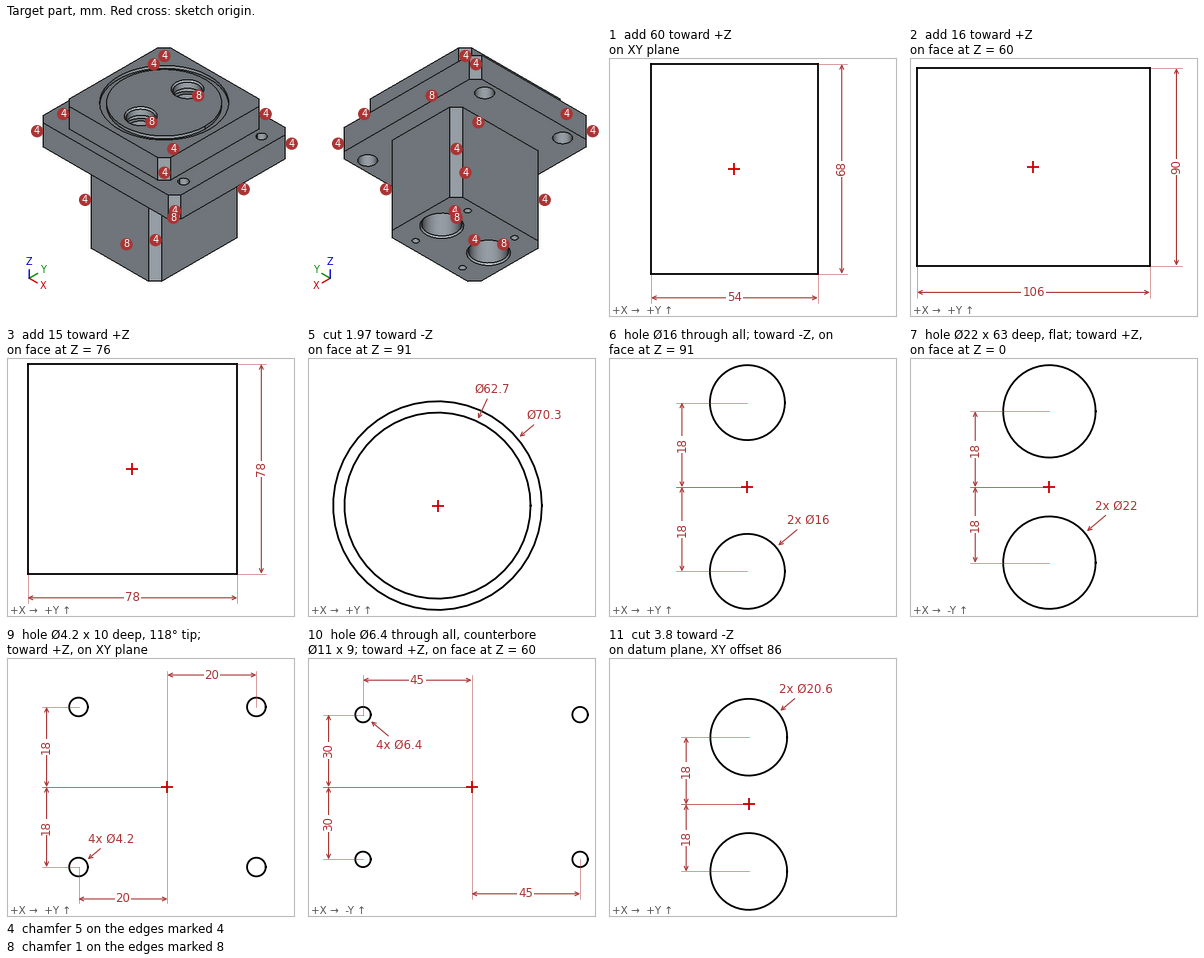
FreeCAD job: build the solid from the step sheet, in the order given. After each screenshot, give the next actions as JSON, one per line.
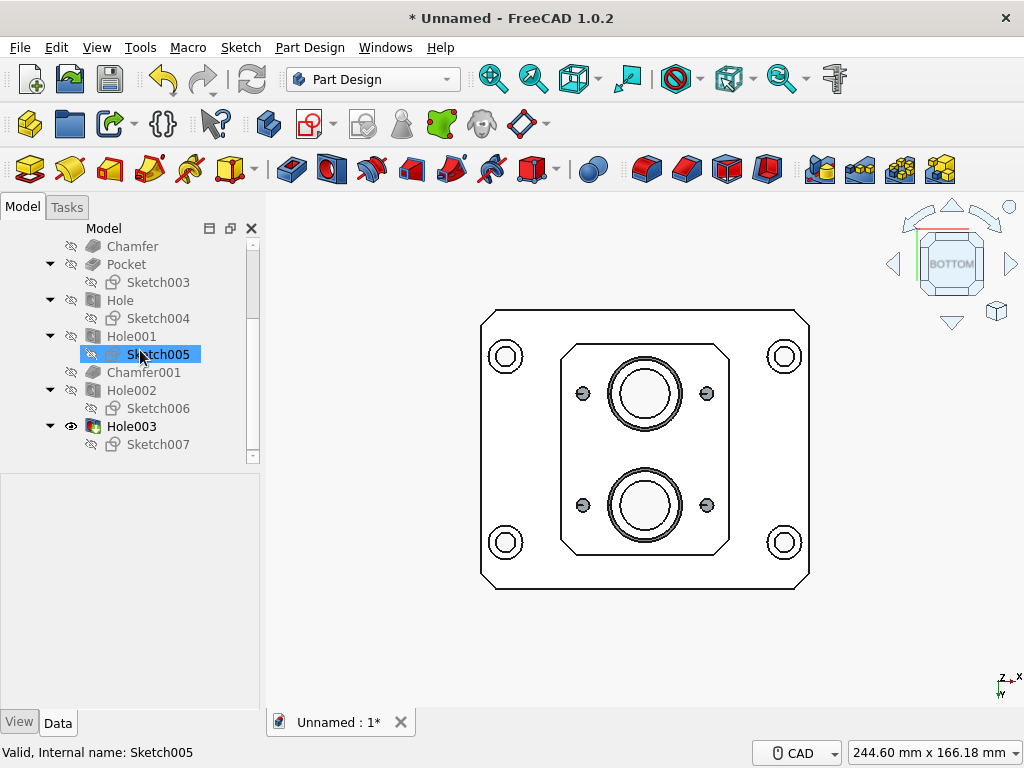
{"action": "scroll", "coordinate": [140, 350], "scroll_direction": "up", "scroll_amount": 15}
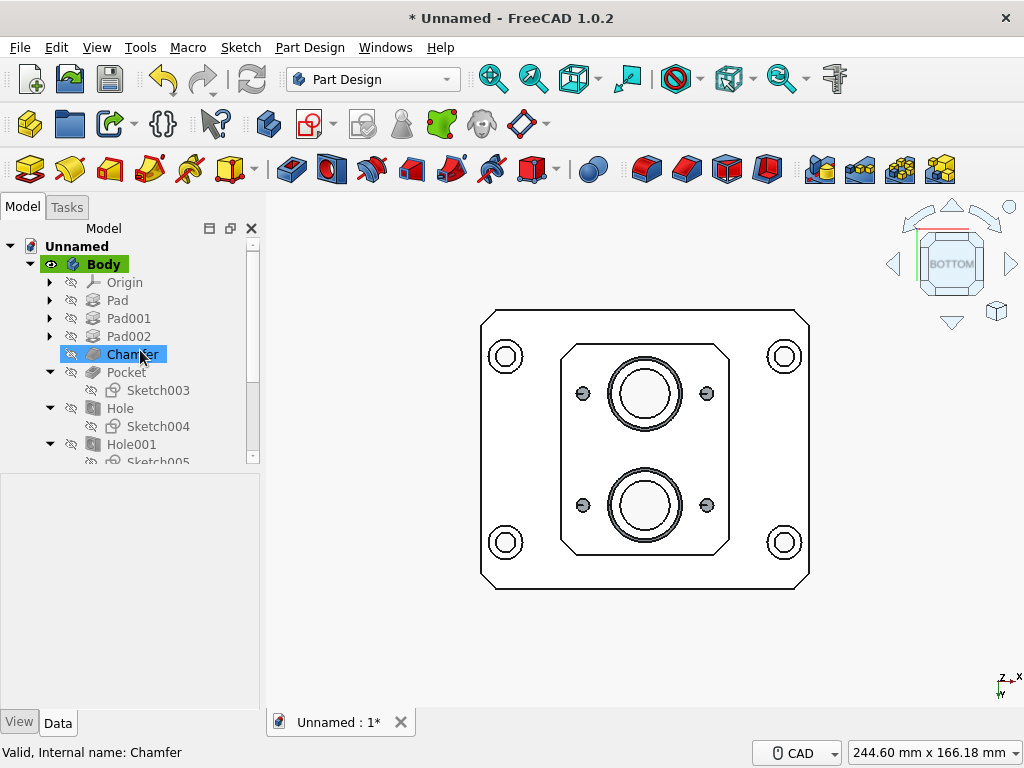
{"action": "left_click", "coordinate": [50, 282]}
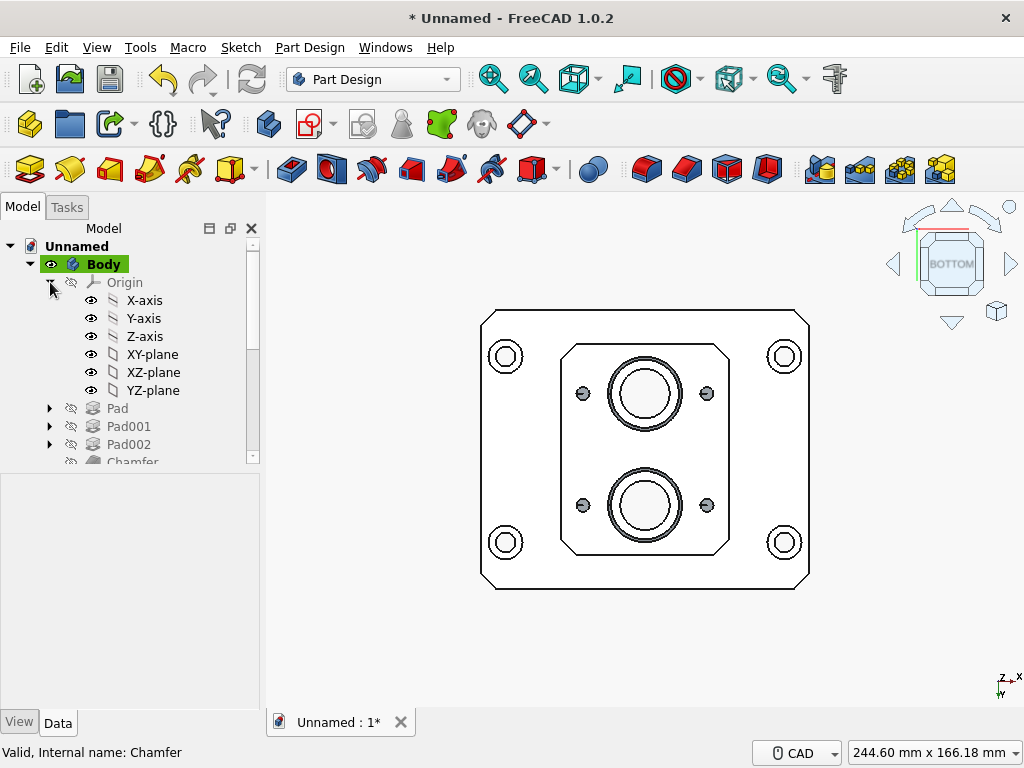
{"action": "left_click", "coordinate": [136, 354]}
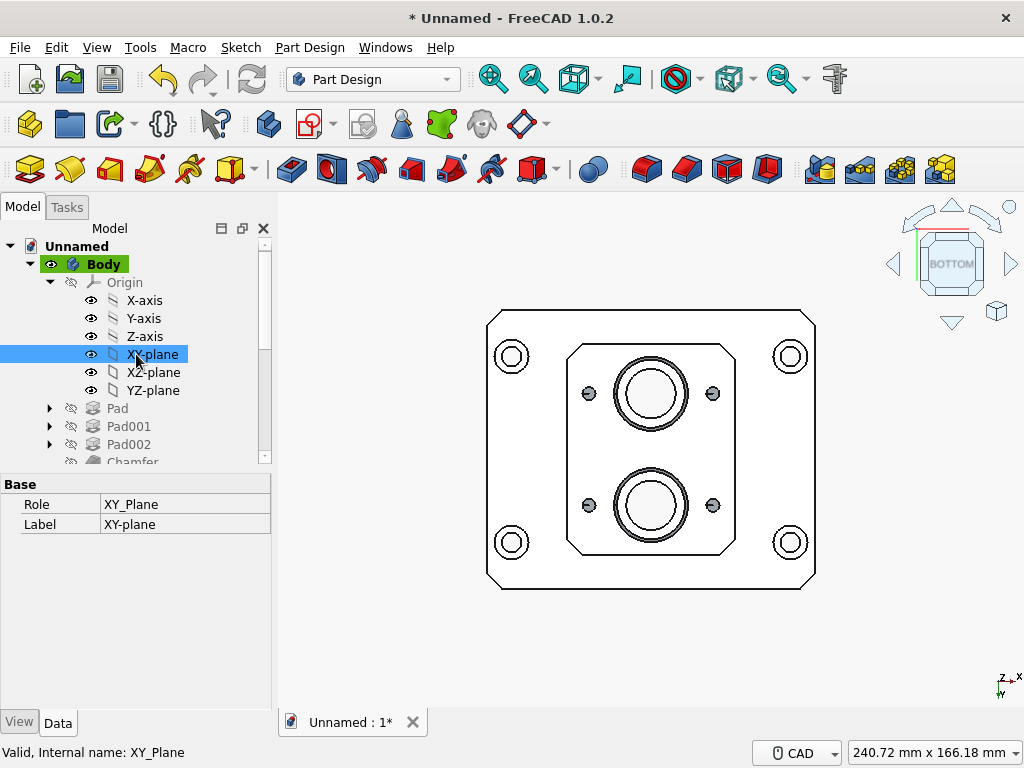
{"action": "left_click", "coordinate": [522, 124]}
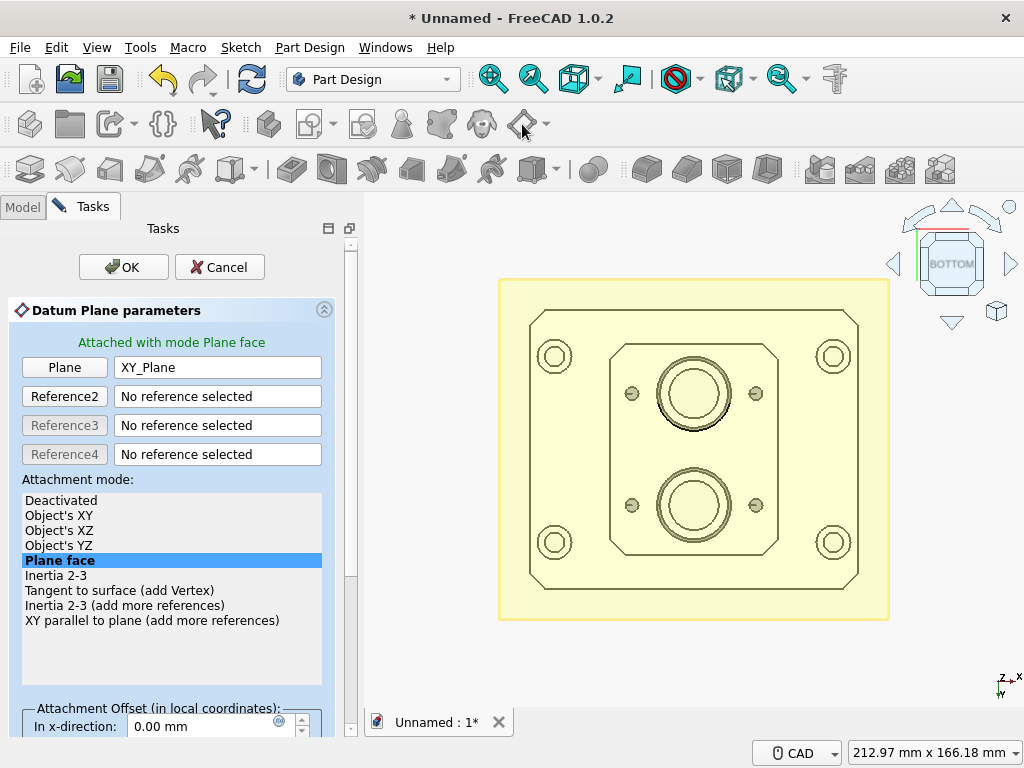
{"action": "scroll", "coordinate": [351, 487], "scroll_direction": "down", "scroll_amount": 3}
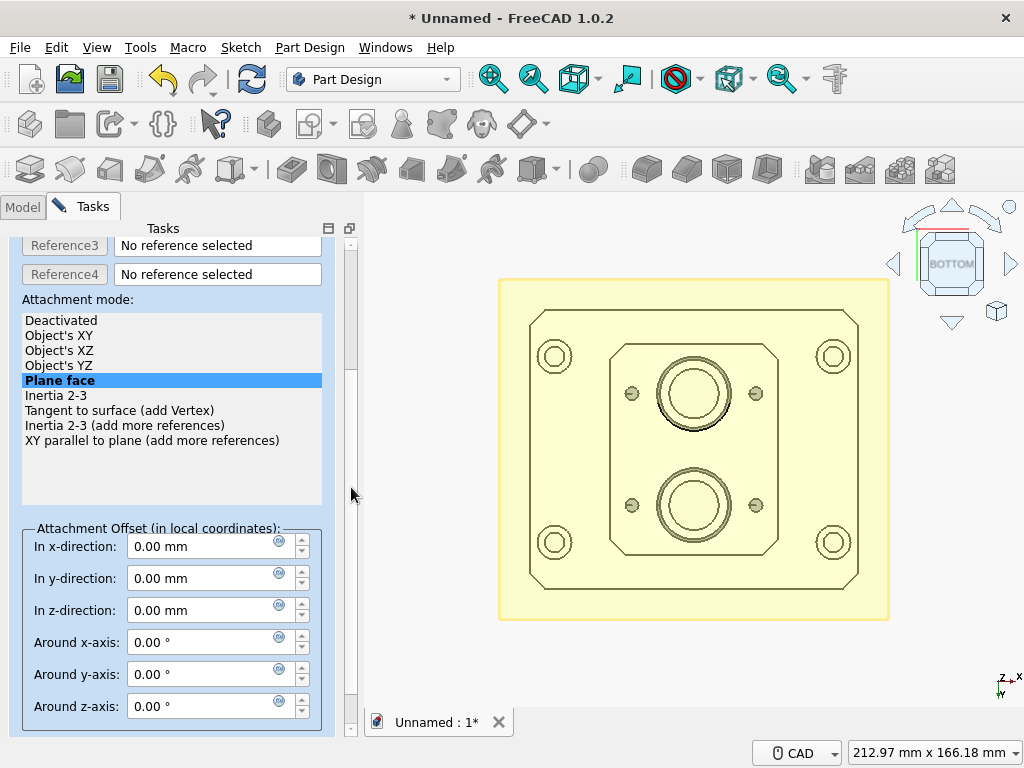
{"action": "triple_click", "coordinate": [210, 610]}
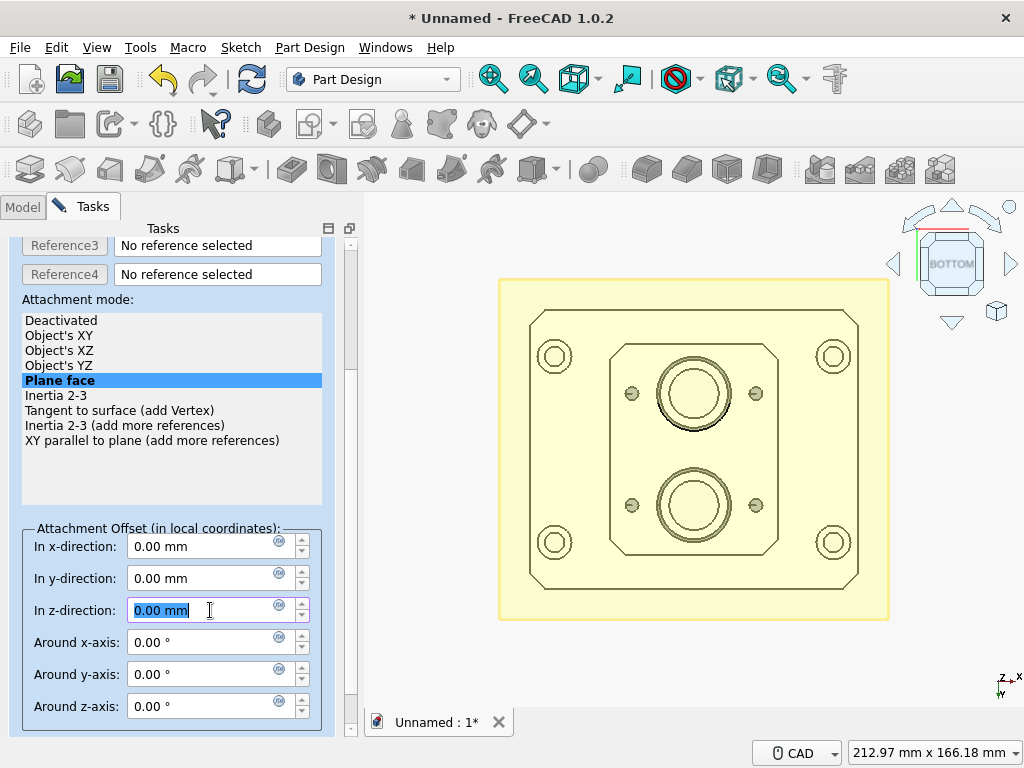
{"action": "type", "text": "86"}
{"action": "key", "text": "Tab"}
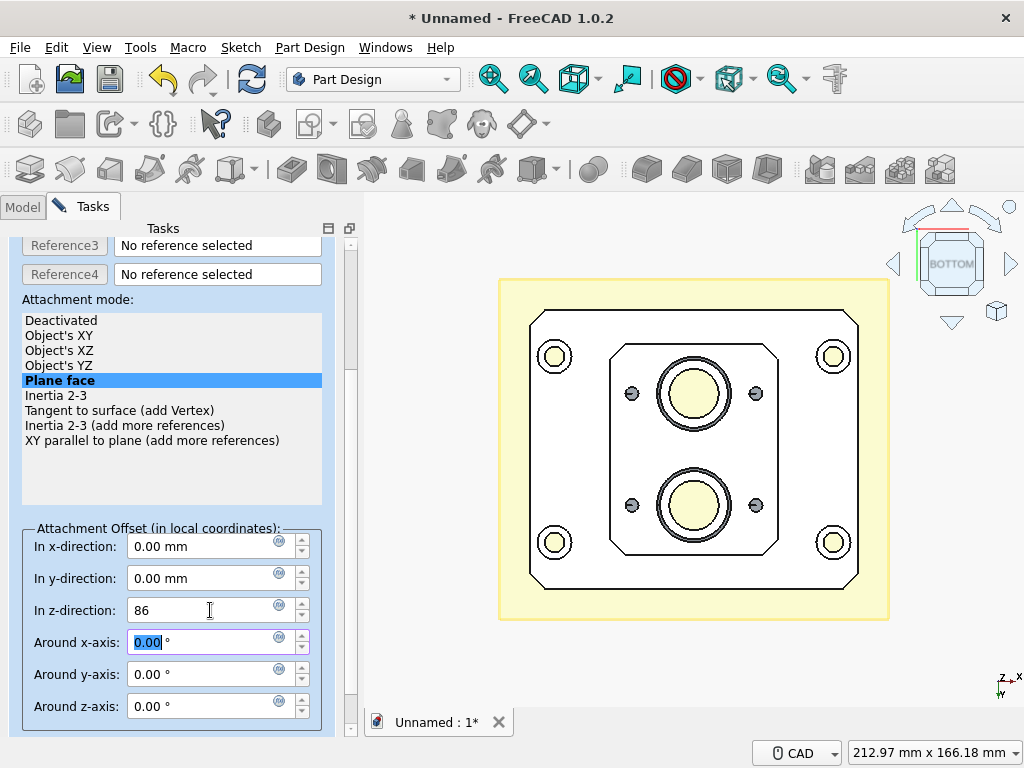
{"action": "scroll", "coordinate": [351, 487], "scroll_direction": "up", "scroll_amount": 4}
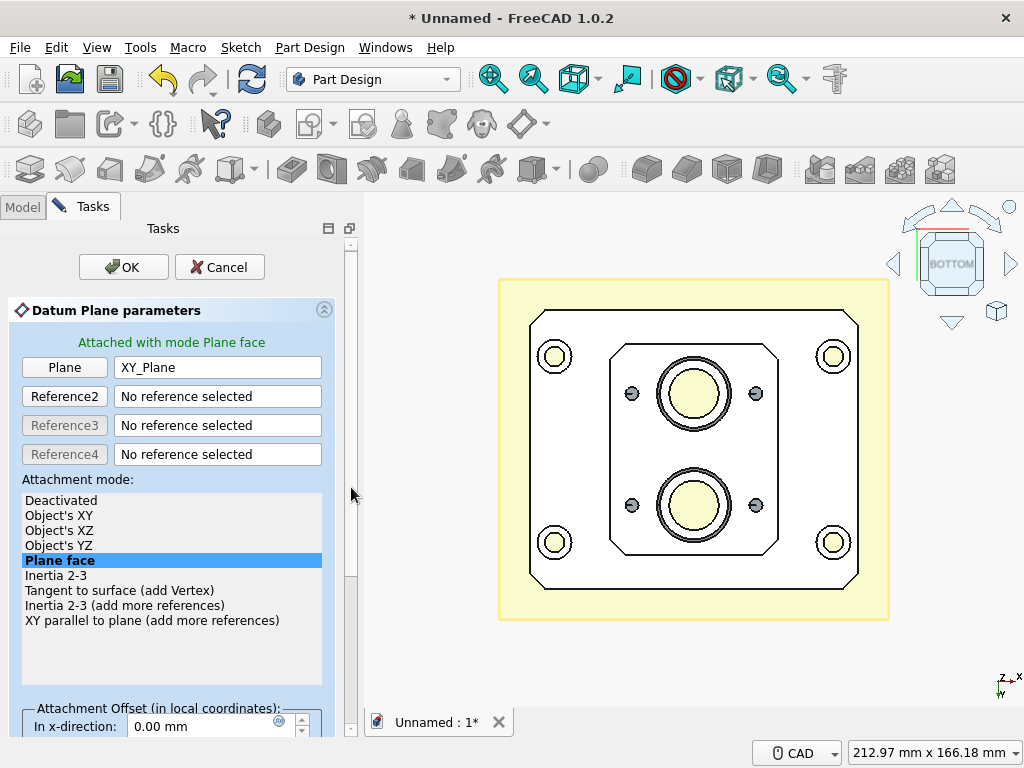
{"action": "left_click", "coordinate": [124, 267]}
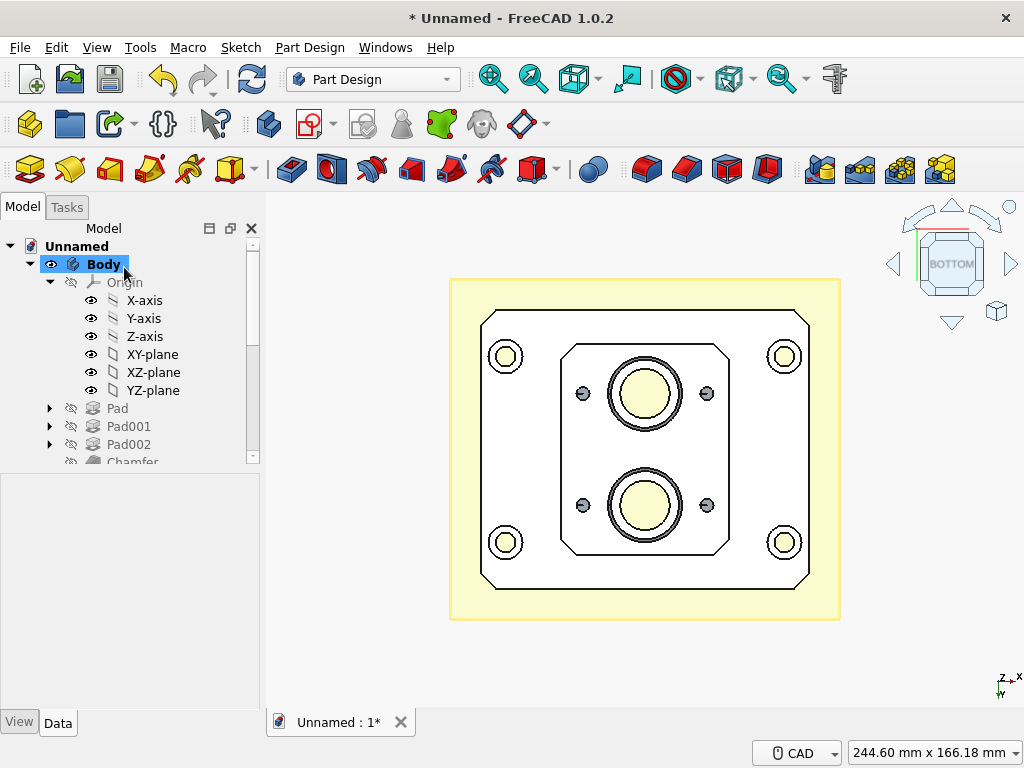
{"action": "scroll", "coordinate": [100, 350], "scroll_direction": "down", "scroll_amount": 3}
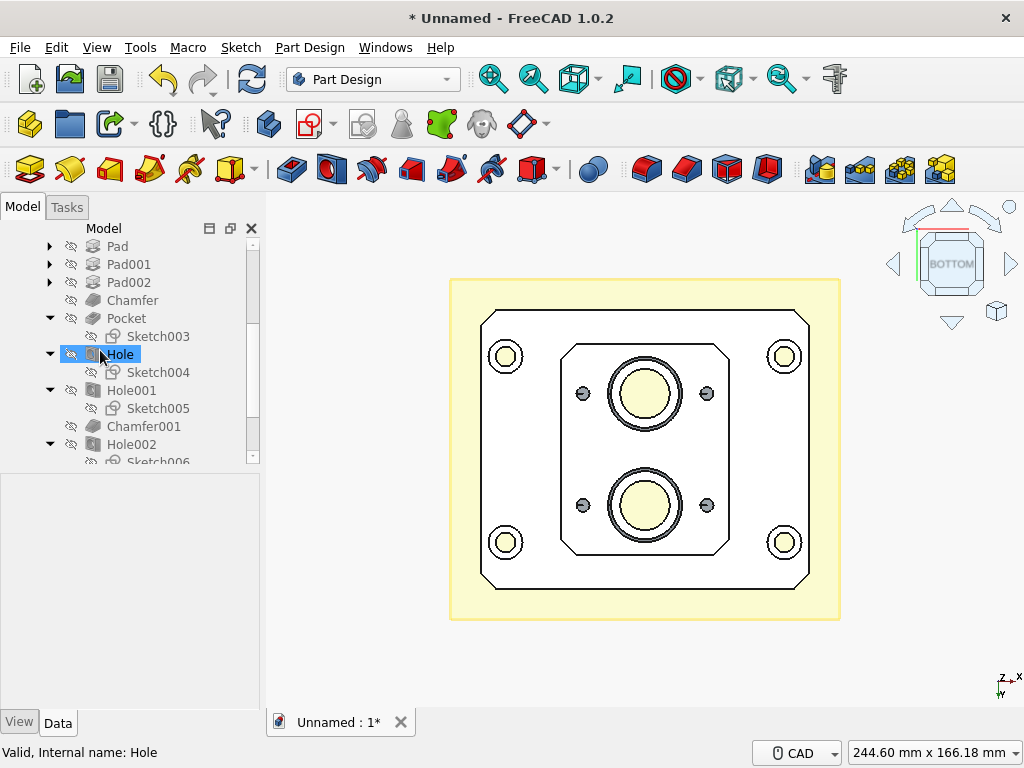
{"action": "scroll", "coordinate": [140, 350], "scroll_direction": "up", "scroll_amount": 15}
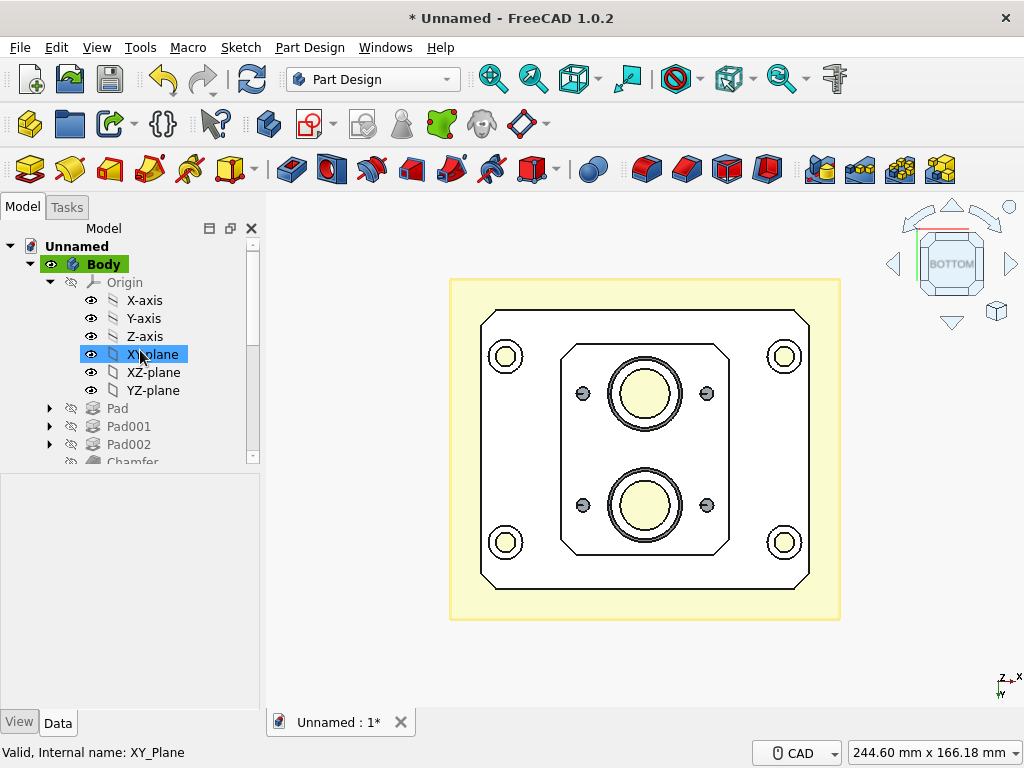
{"action": "scroll", "coordinate": [100, 350], "scroll_direction": "down", "scroll_amount": 6}